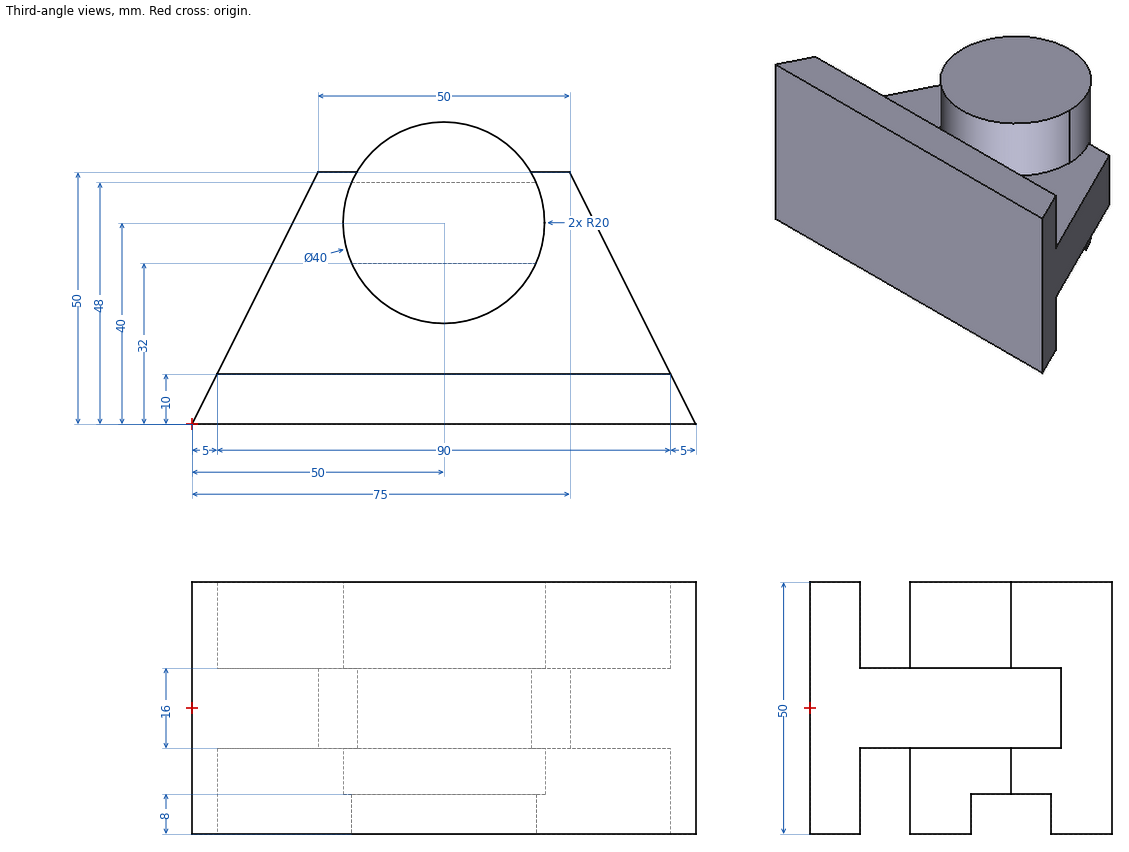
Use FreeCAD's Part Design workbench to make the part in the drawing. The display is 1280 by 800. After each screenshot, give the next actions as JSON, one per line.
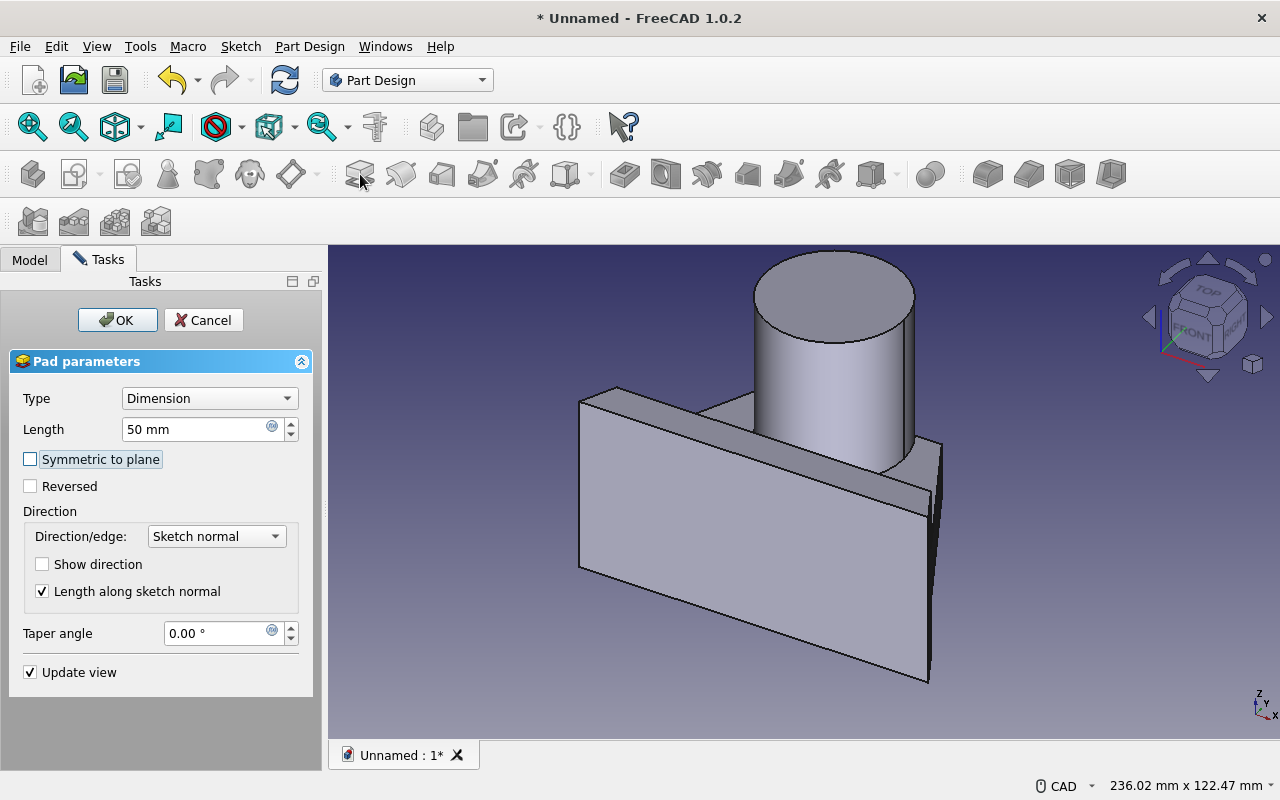
{"action": "left_click", "coordinate": [31, 459]}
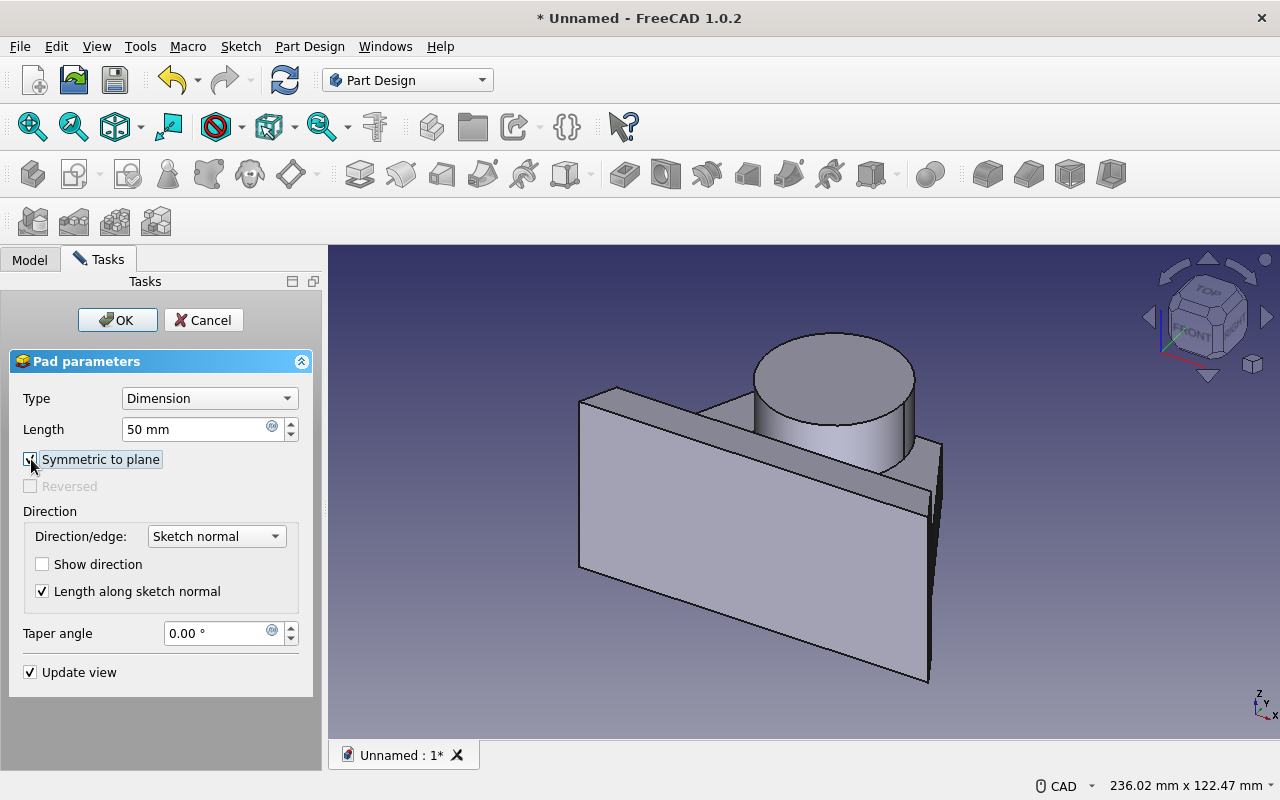
{"action": "left_click", "coordinate": [118, 320]}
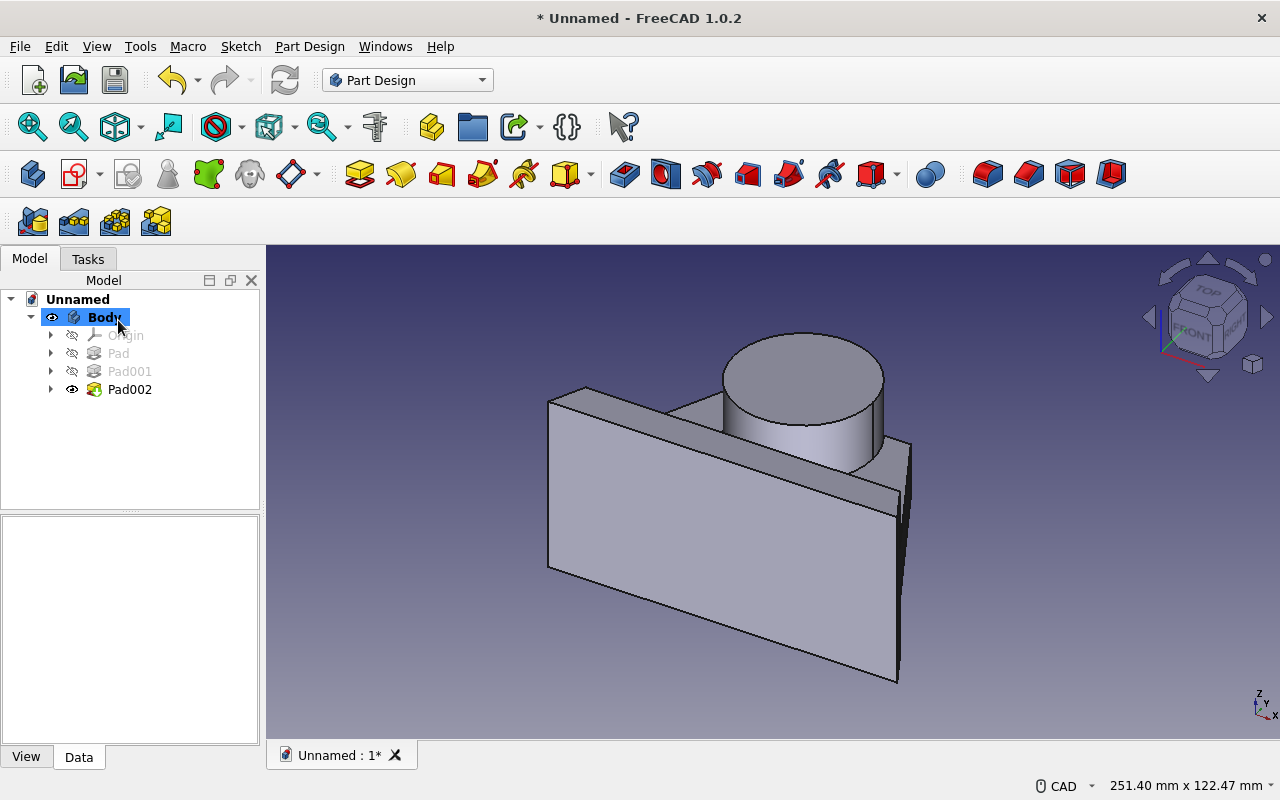
{"action": "left_click", "coordinate": [51, 335]}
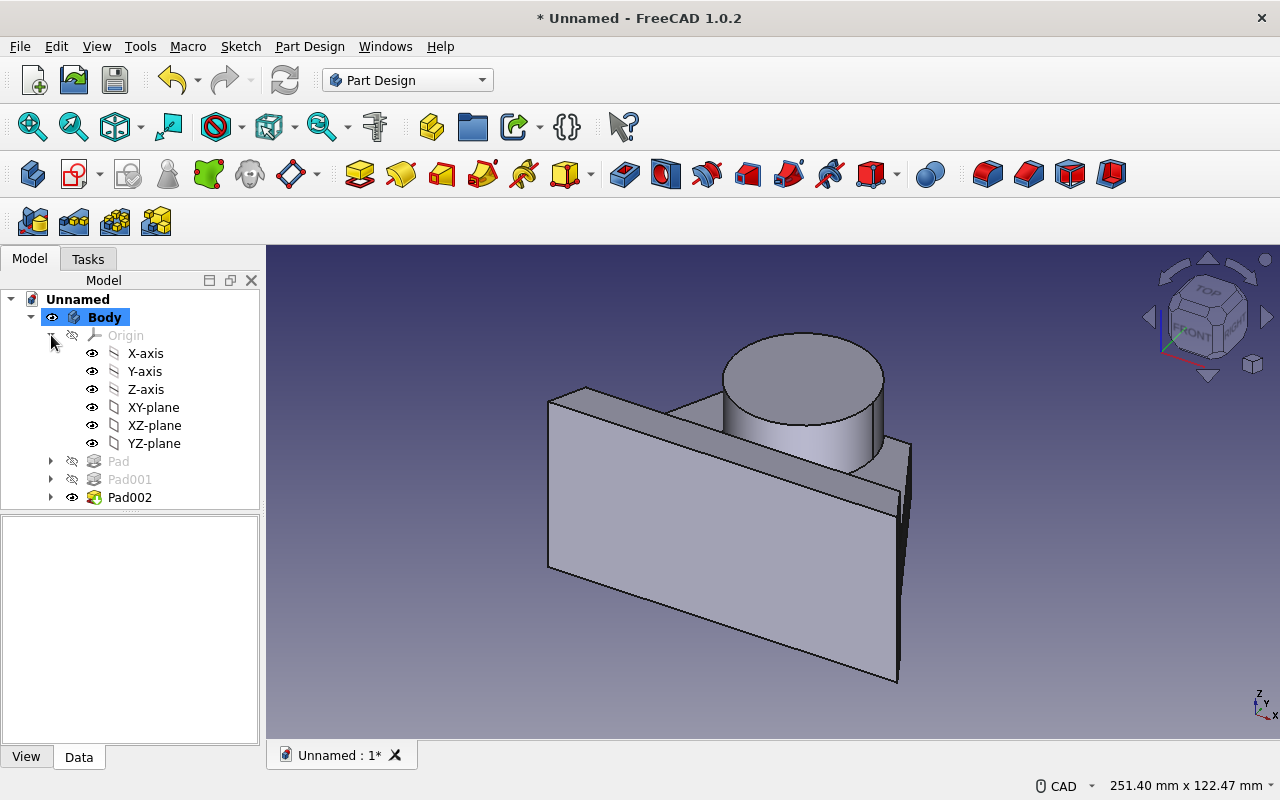
{"action": "left_click", "coordinate": [137, 407]}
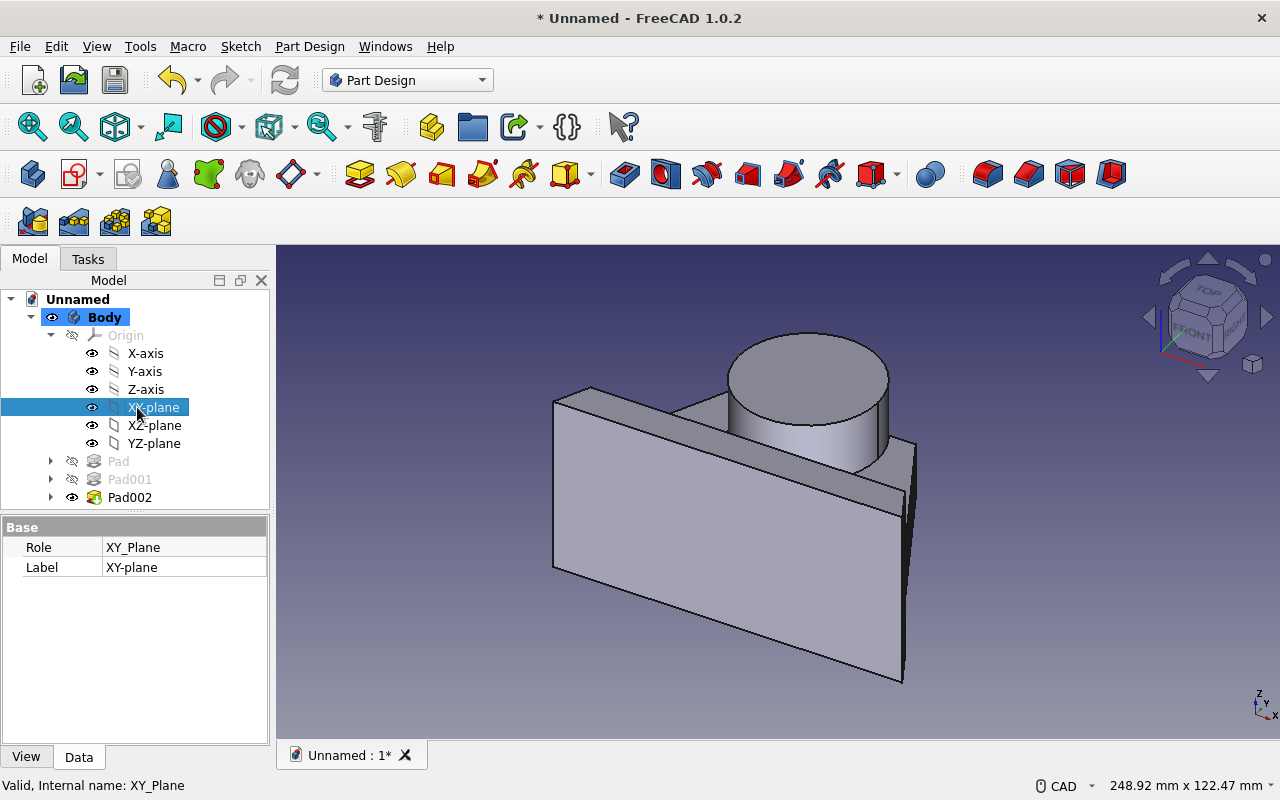
{"action": "left_click", "coordinate": [290, 174]}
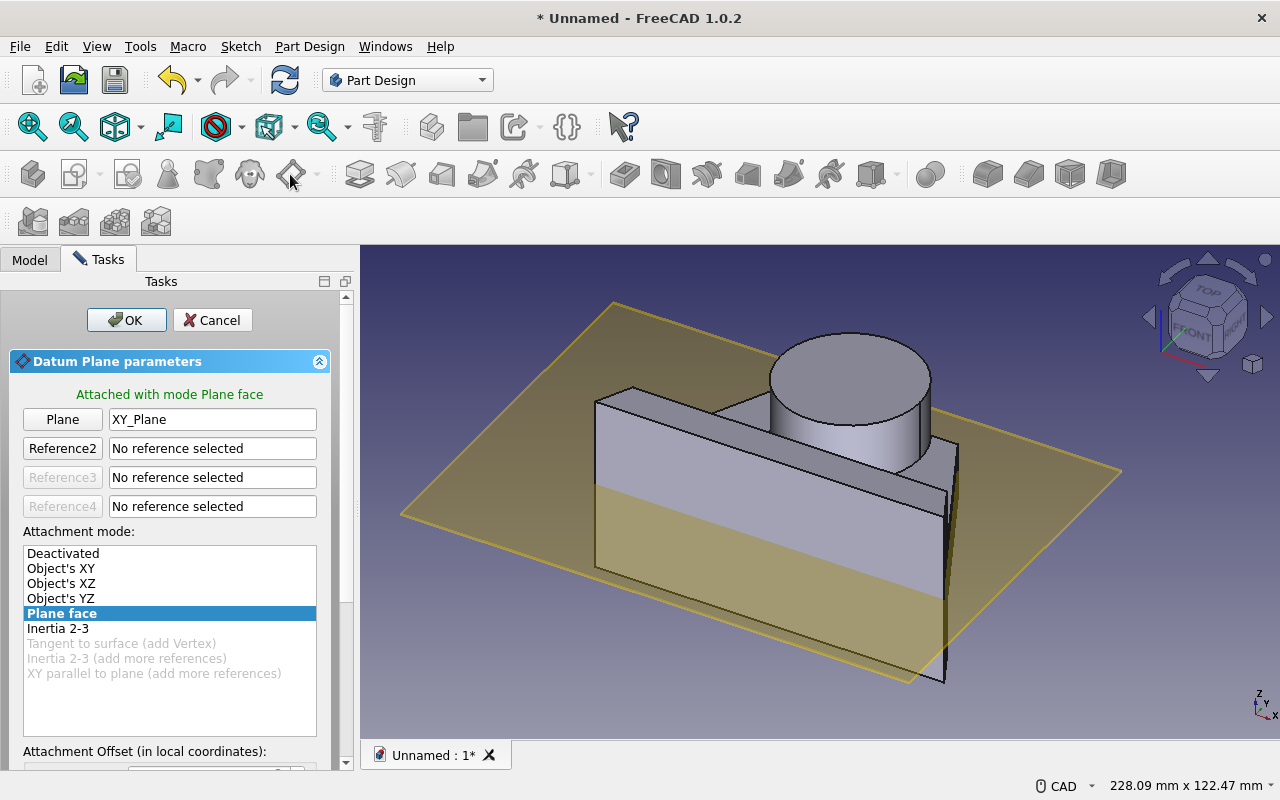
{"action": "scroll", "coordinate": [346, 530], "scroll_direction": "down", "scroll_amount": 3}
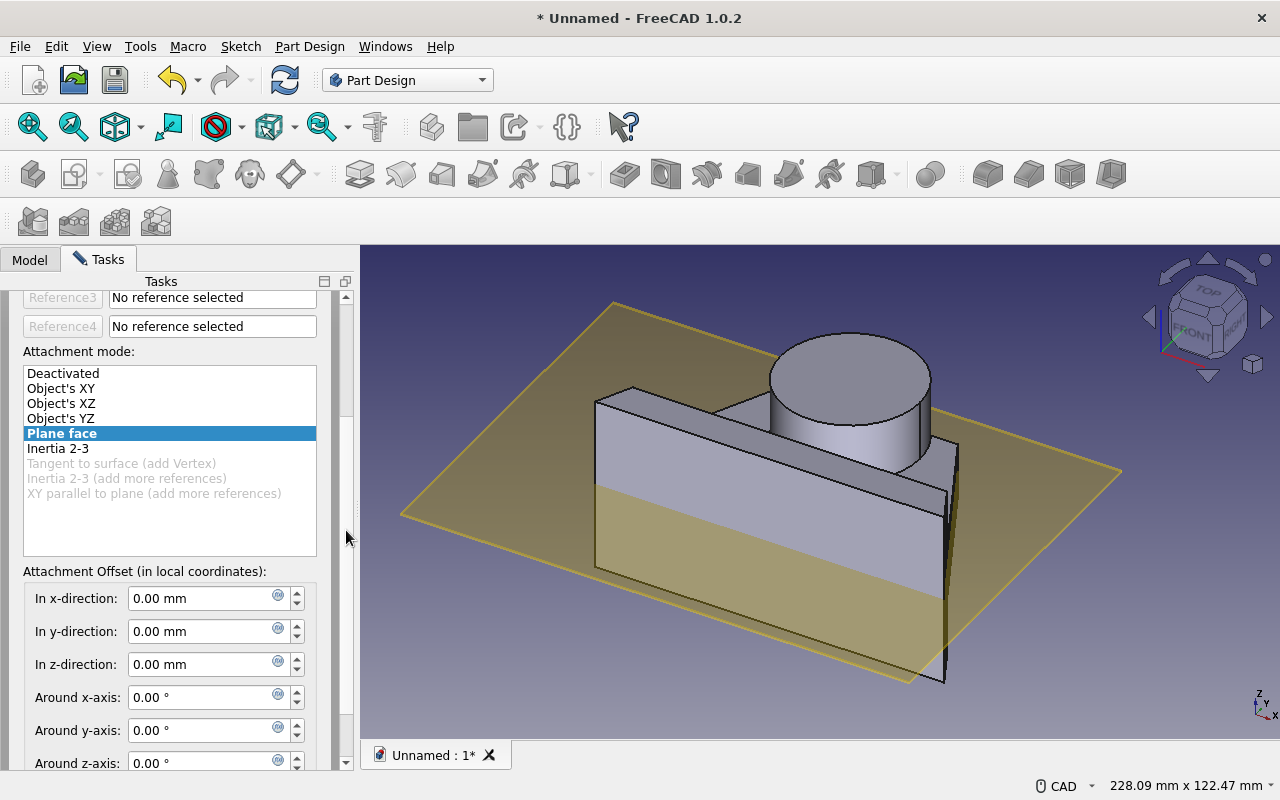
{"action": "triple_click", "coordinate": [210, 664]}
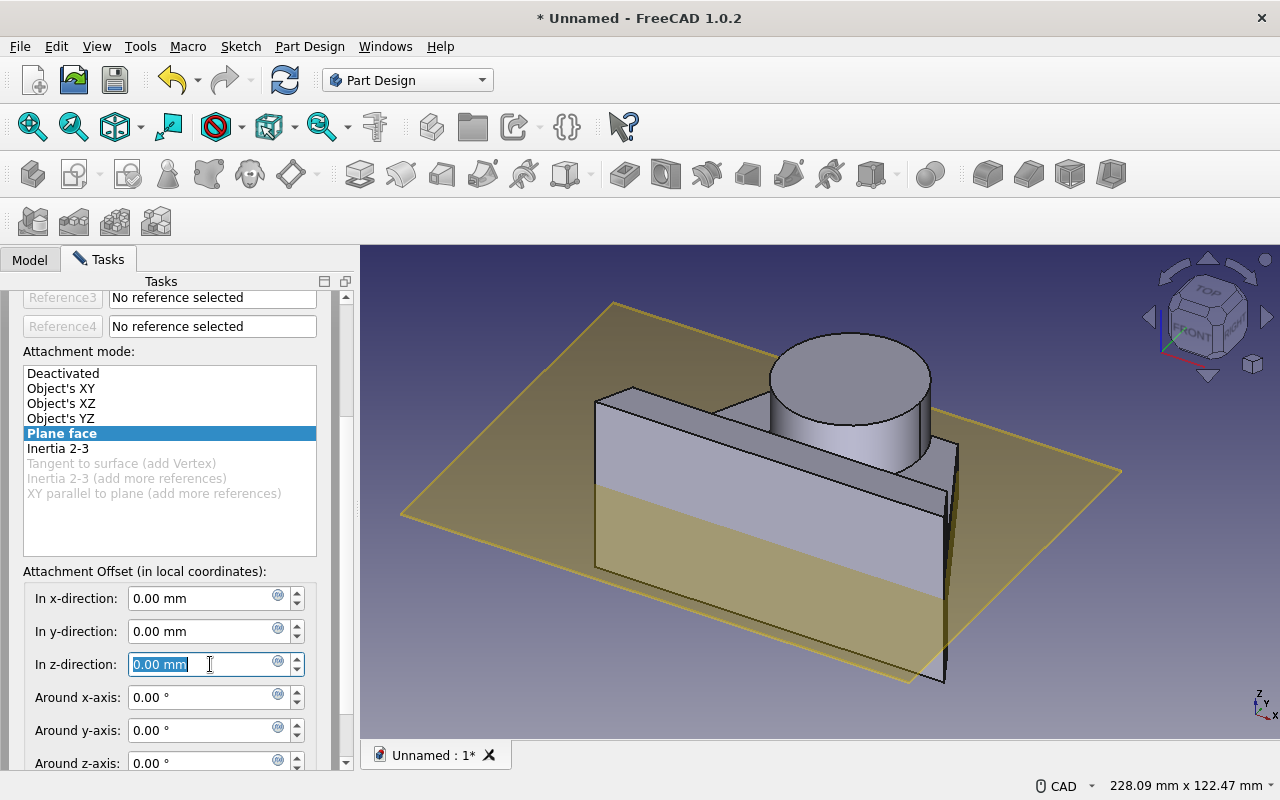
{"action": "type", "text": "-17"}
{"action": "key", "text": "Tab"}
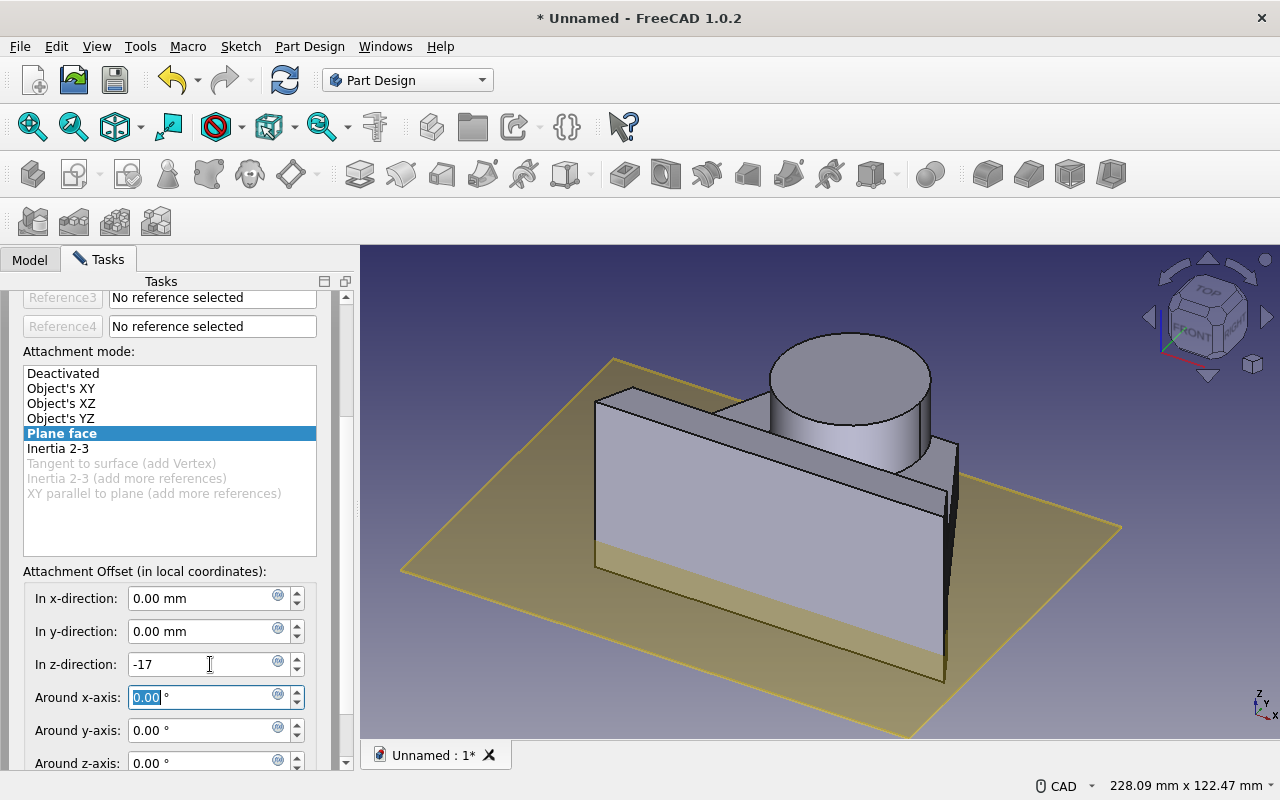
{"action": "scroll", "coordinate": [346, 530], "scroll_direction": "up", "scroll_amount": 4}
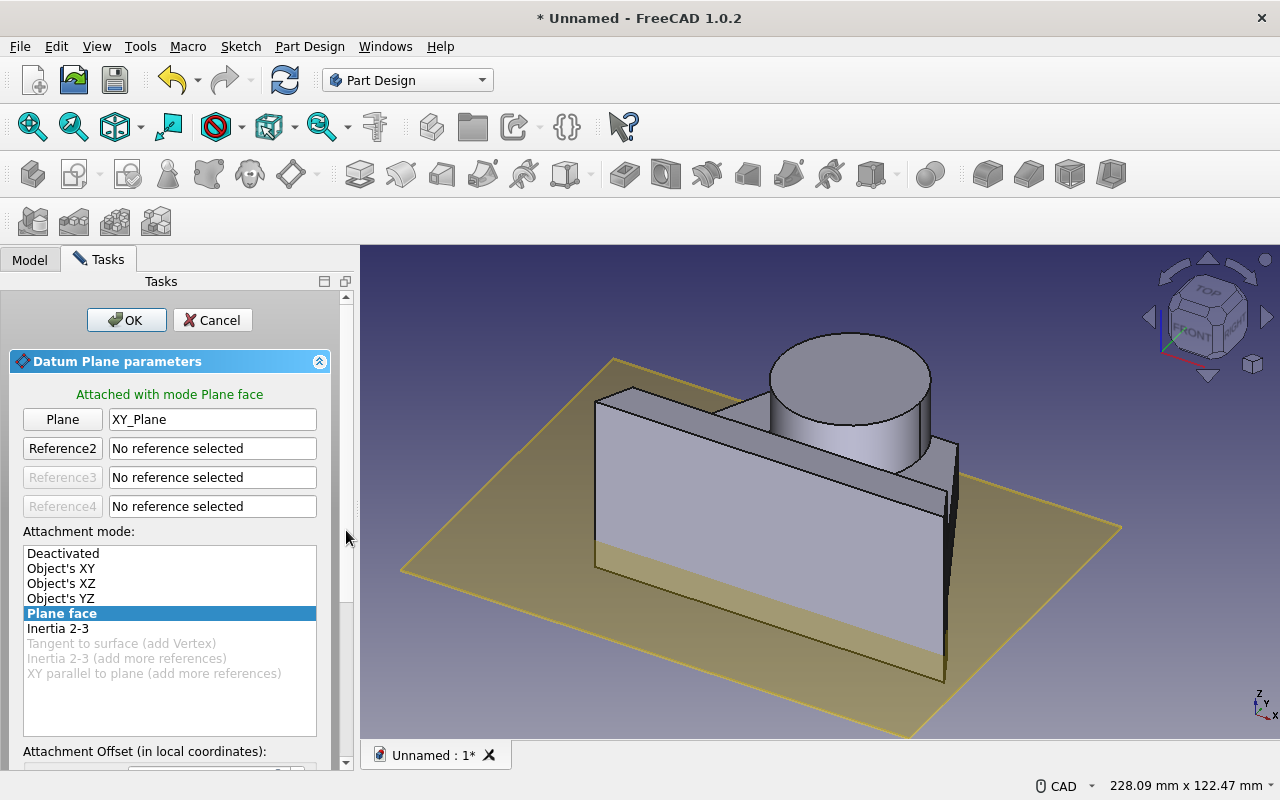
{"action": "left_click", "coordinate": [127, 320]}